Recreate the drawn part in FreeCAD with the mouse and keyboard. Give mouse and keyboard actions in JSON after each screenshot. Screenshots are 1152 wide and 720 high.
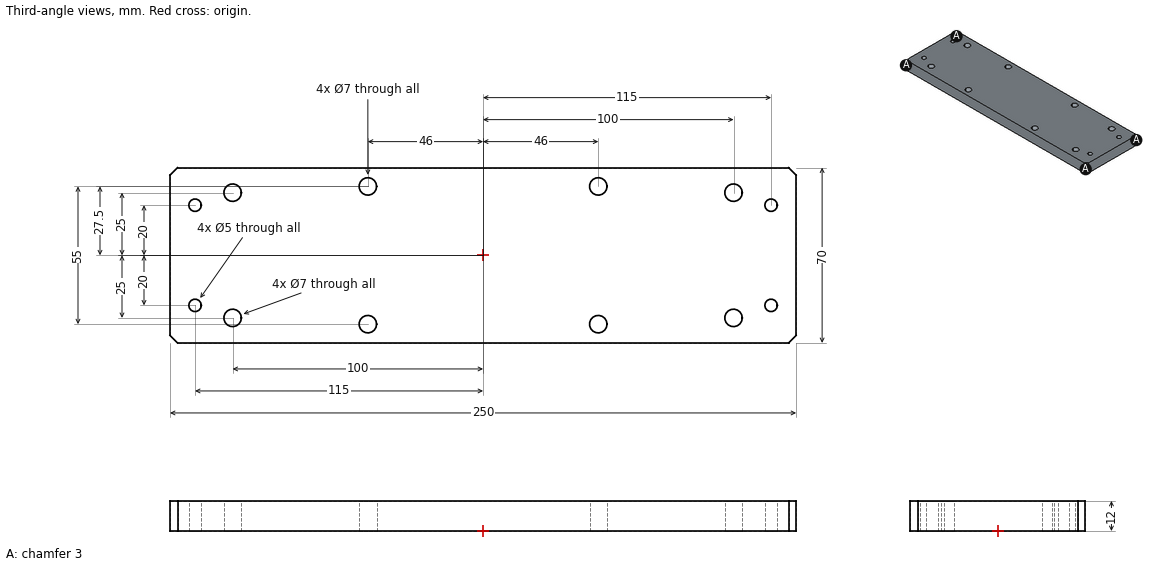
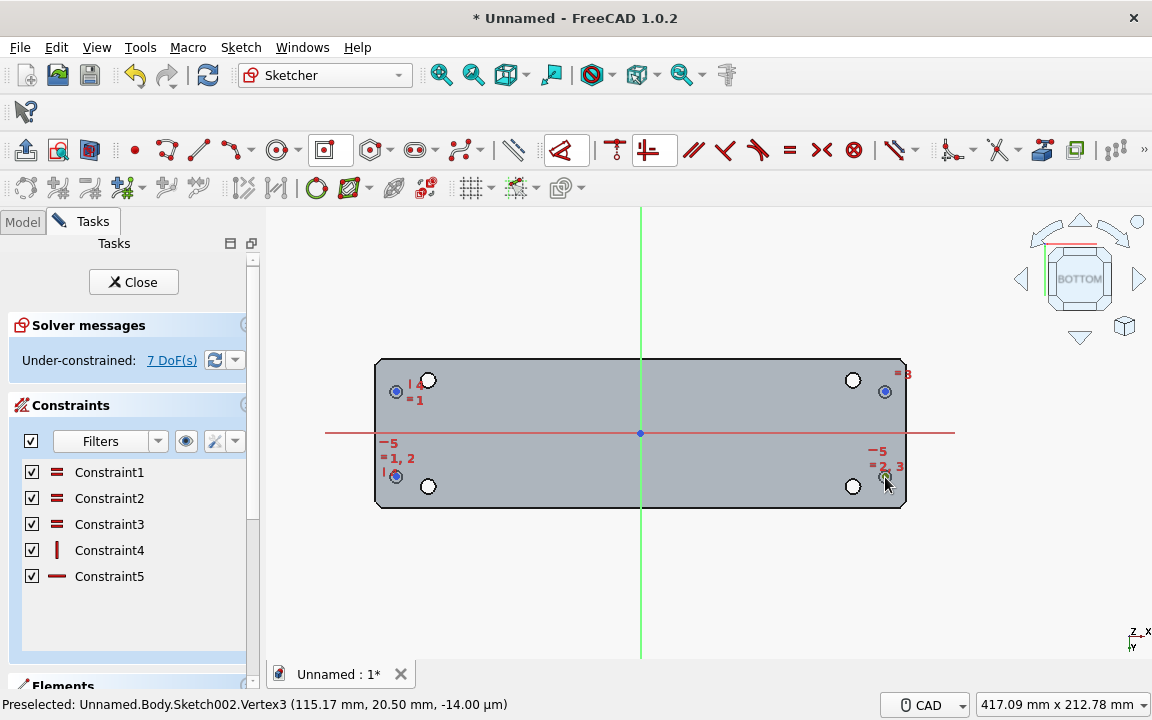
{"action": "left_click", "coordinate": [885, 392]}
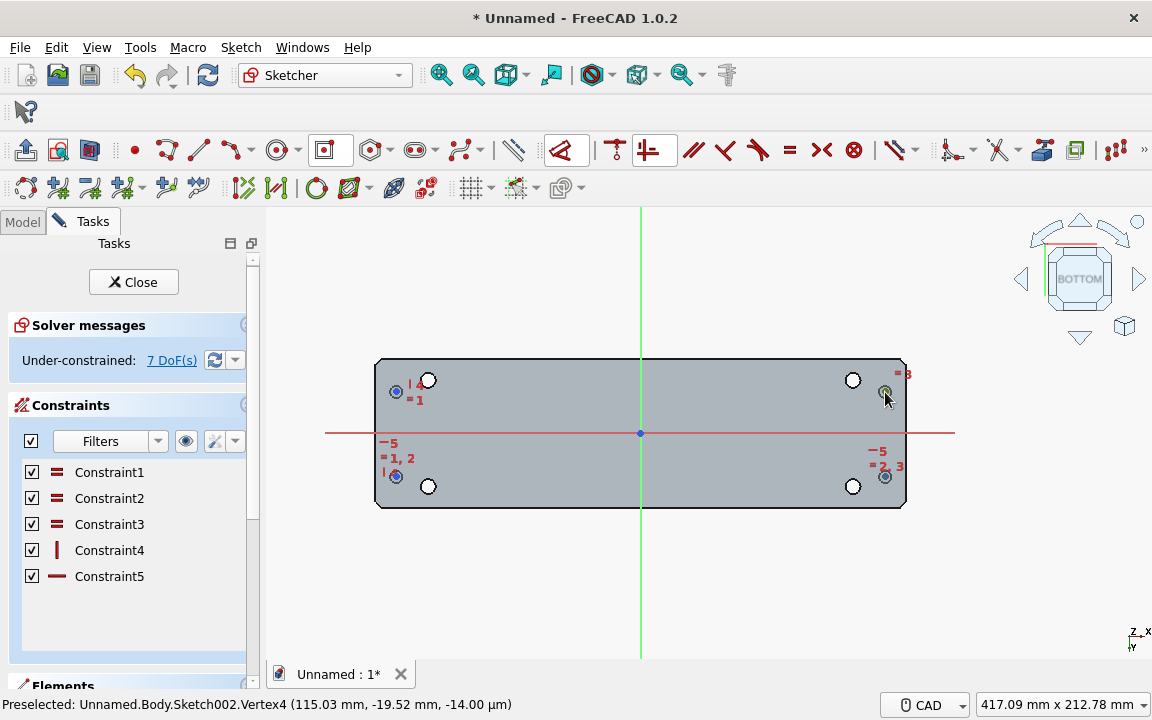
{"action": "left_click", "coordinate": [672, 150]}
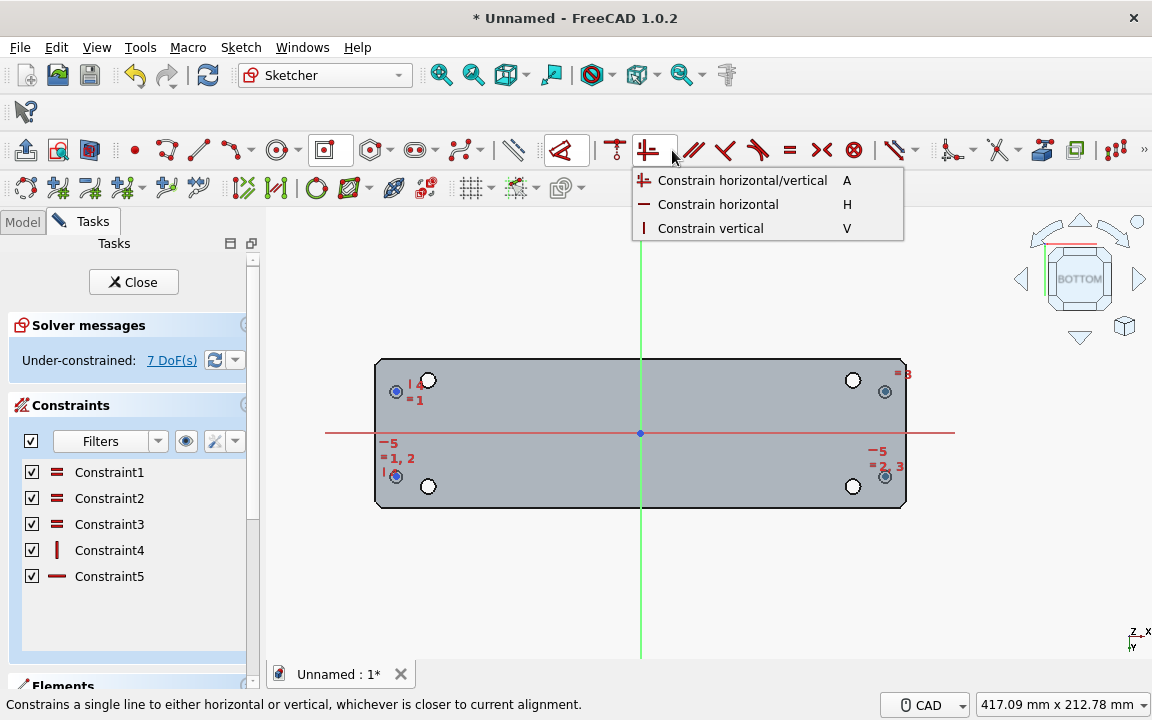
{"action": "left_click", "coordinate": [768, 228]}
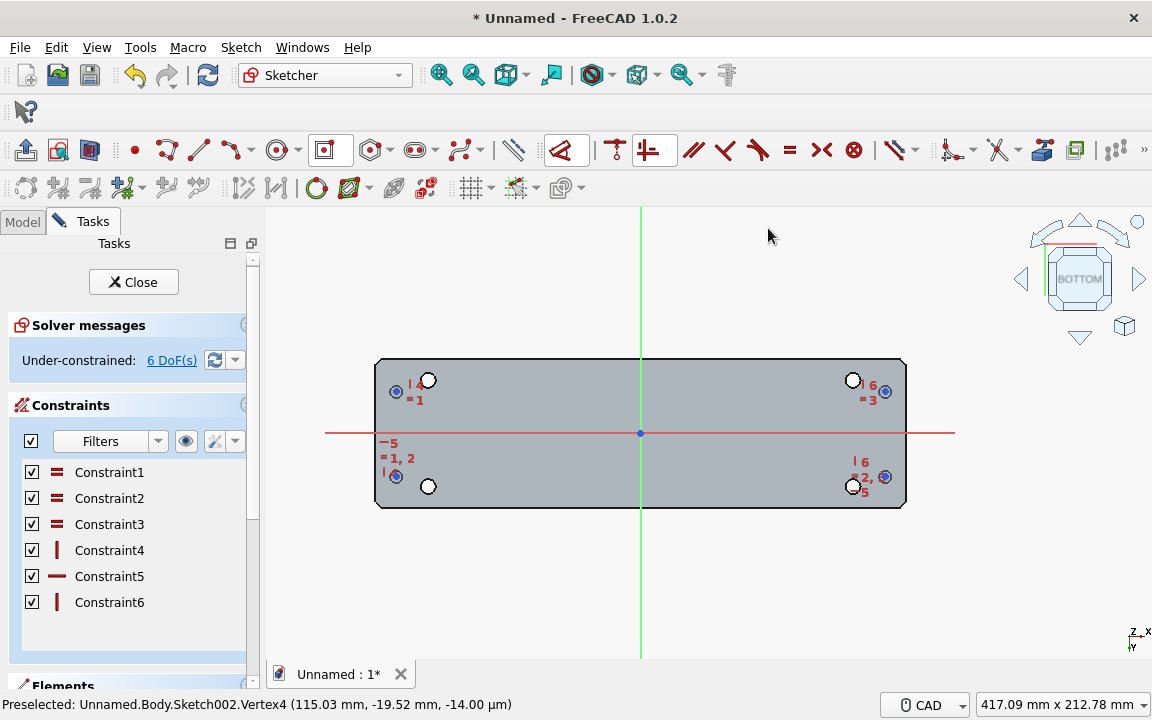
{"action": "left_click", "coordinate": [396, 392]}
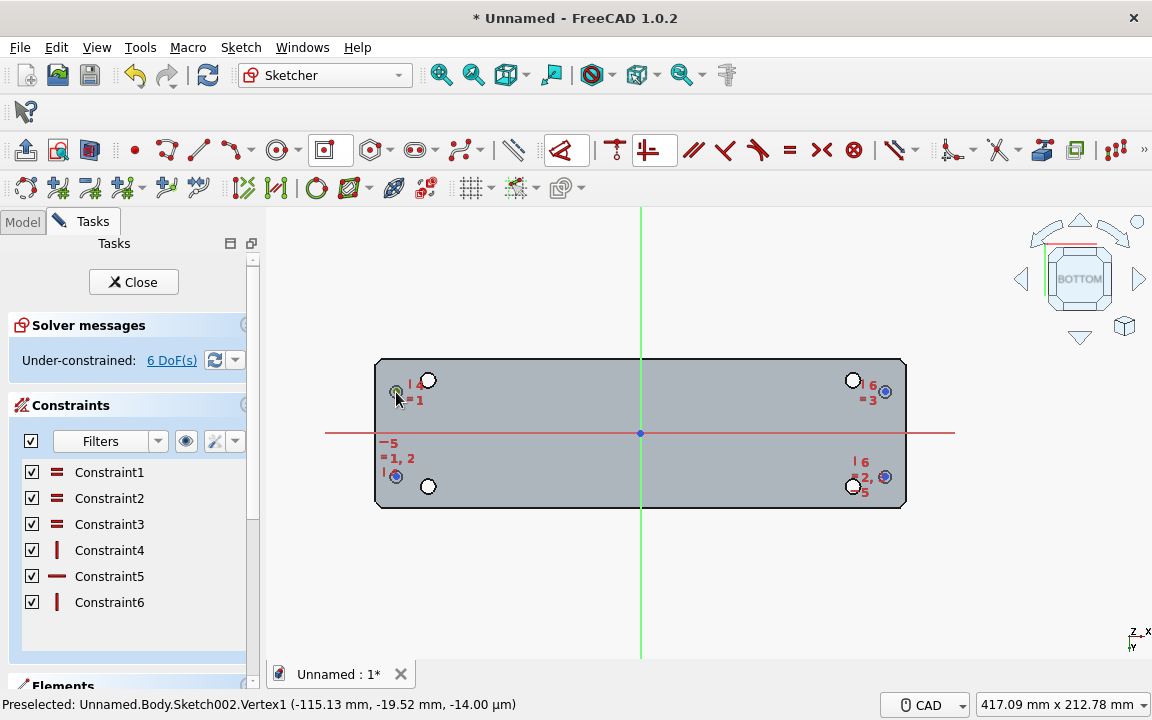
{"action": "left_click", "coordinate": [885, 392]}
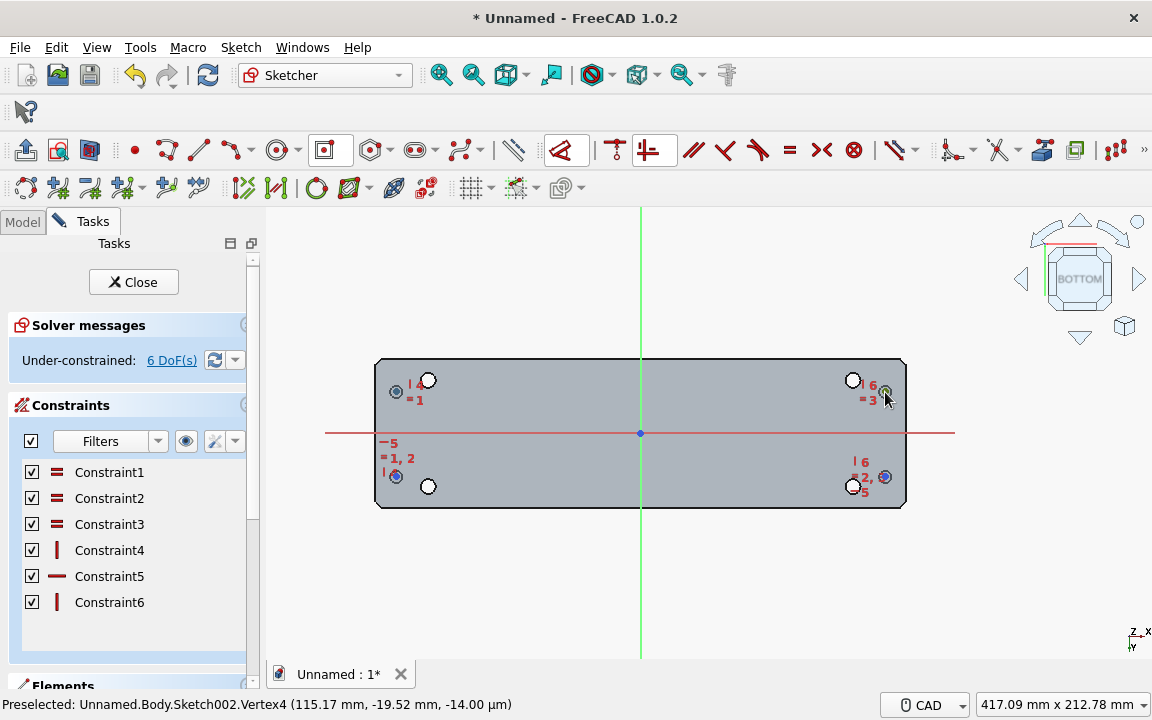
{"action": "key", "text": "h"}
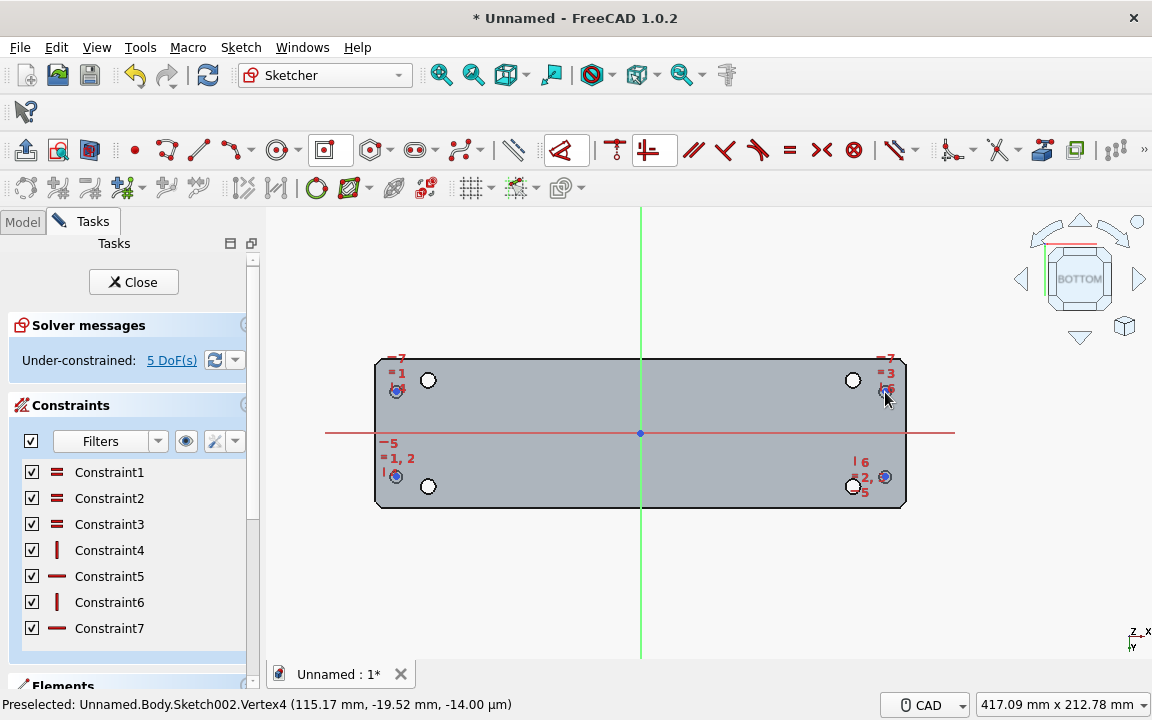
{"action": "scroll", "coordinate": [392, 388], "scroll_direction": "up", "scroll_amount": 7}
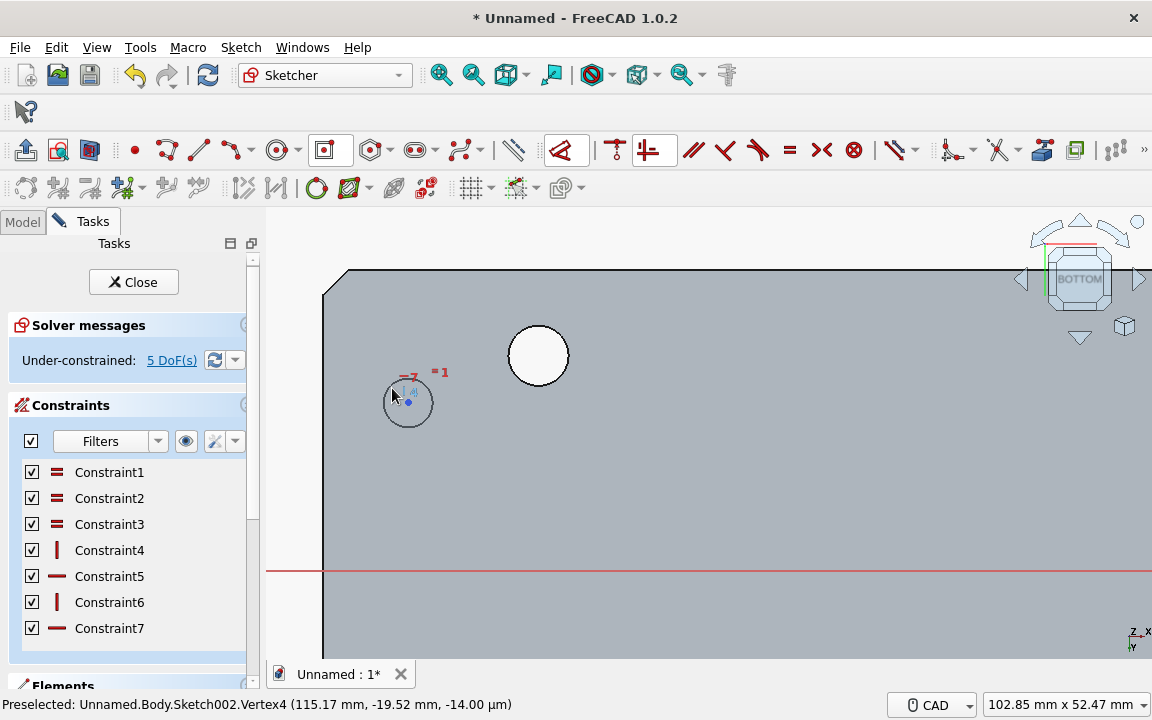
{"action": "left_click", "coordinate": [391, 386]}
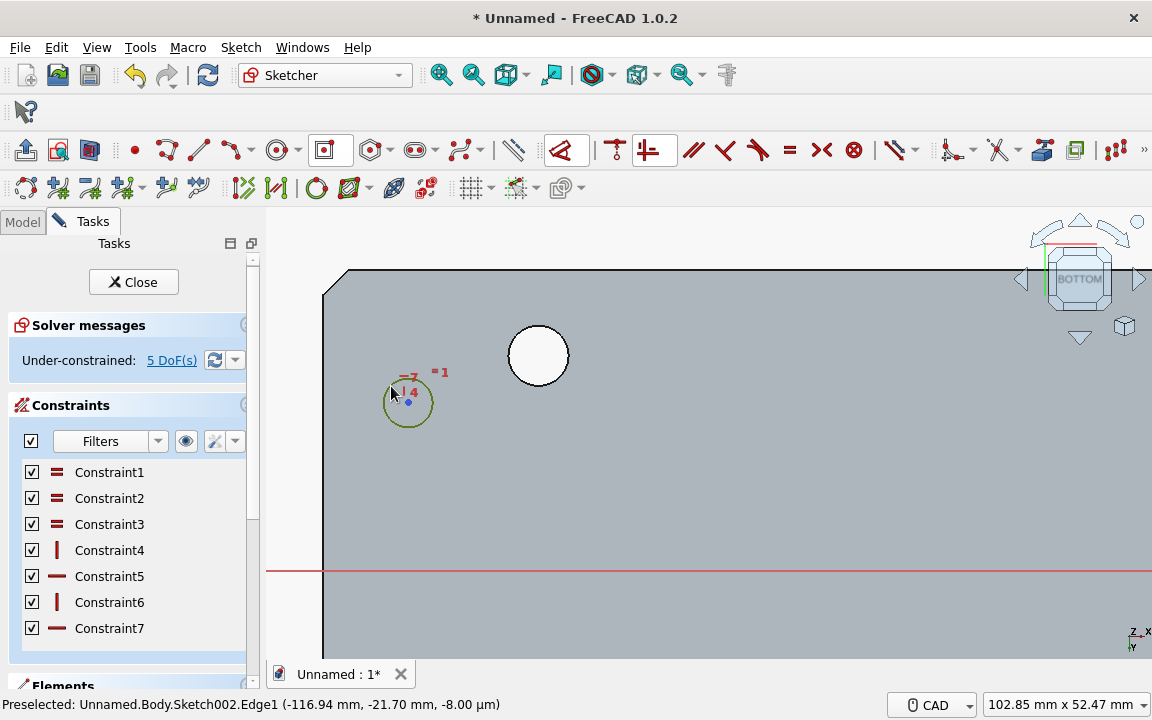
{"action": "left_click", "coordinate": [584, 150]}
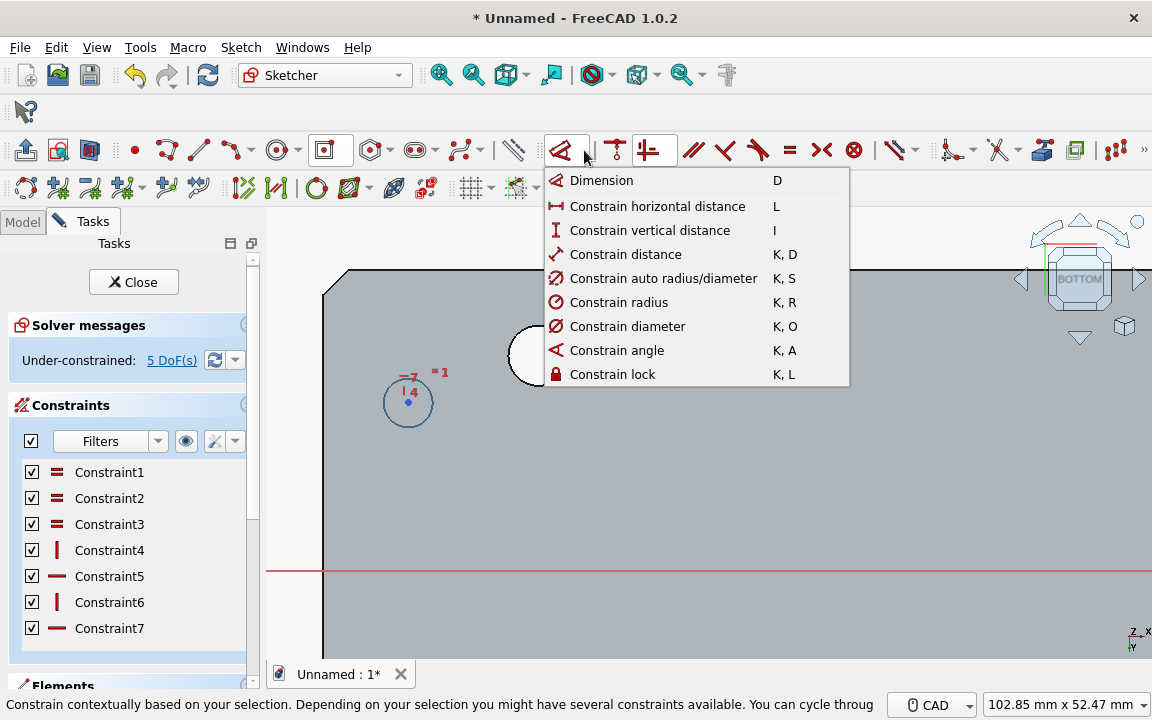
{"action": "left_click", "coordinate": [697, 326]}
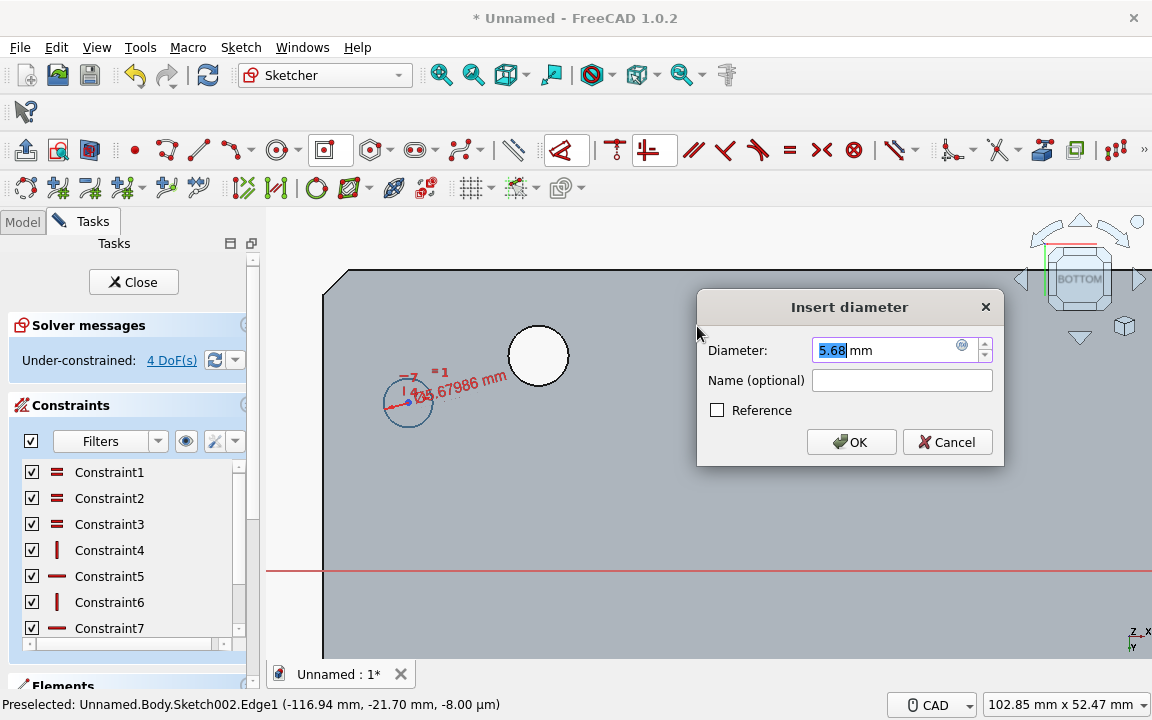
{"action": "type", "text": "5"}
{"action": "key", "text": "Return"}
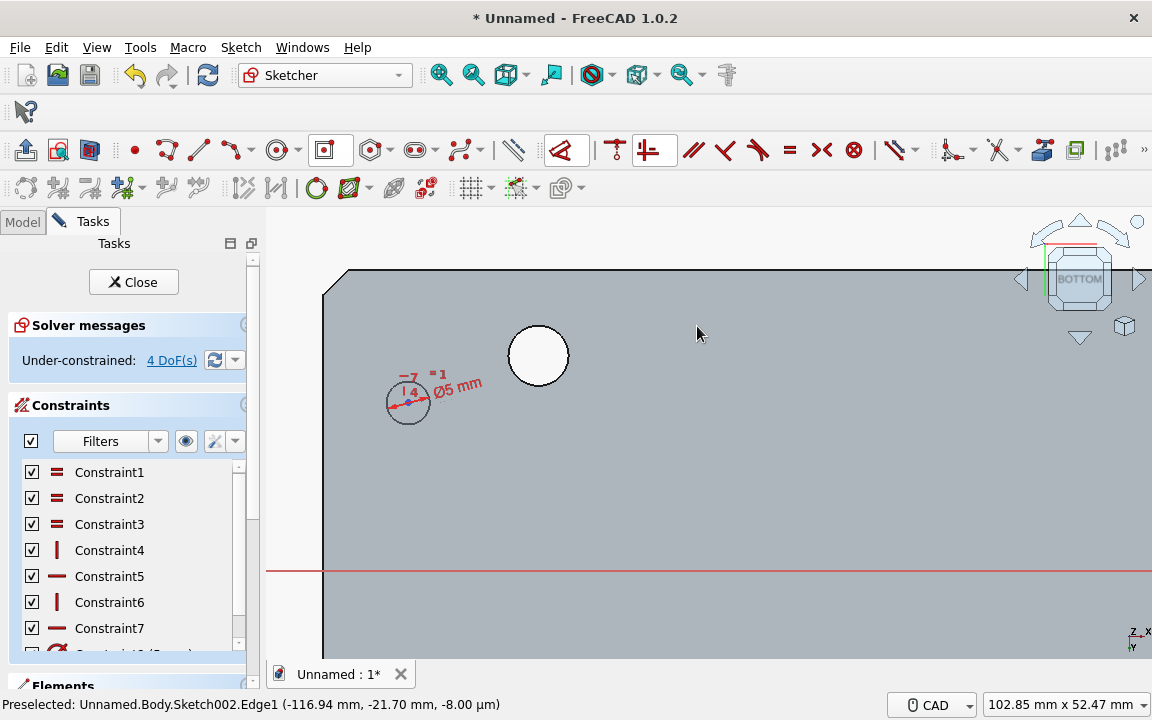
{"action": "scroll", "coordinate": [392, 388], "scroll_direction": "down", "scroll_amount": 7}